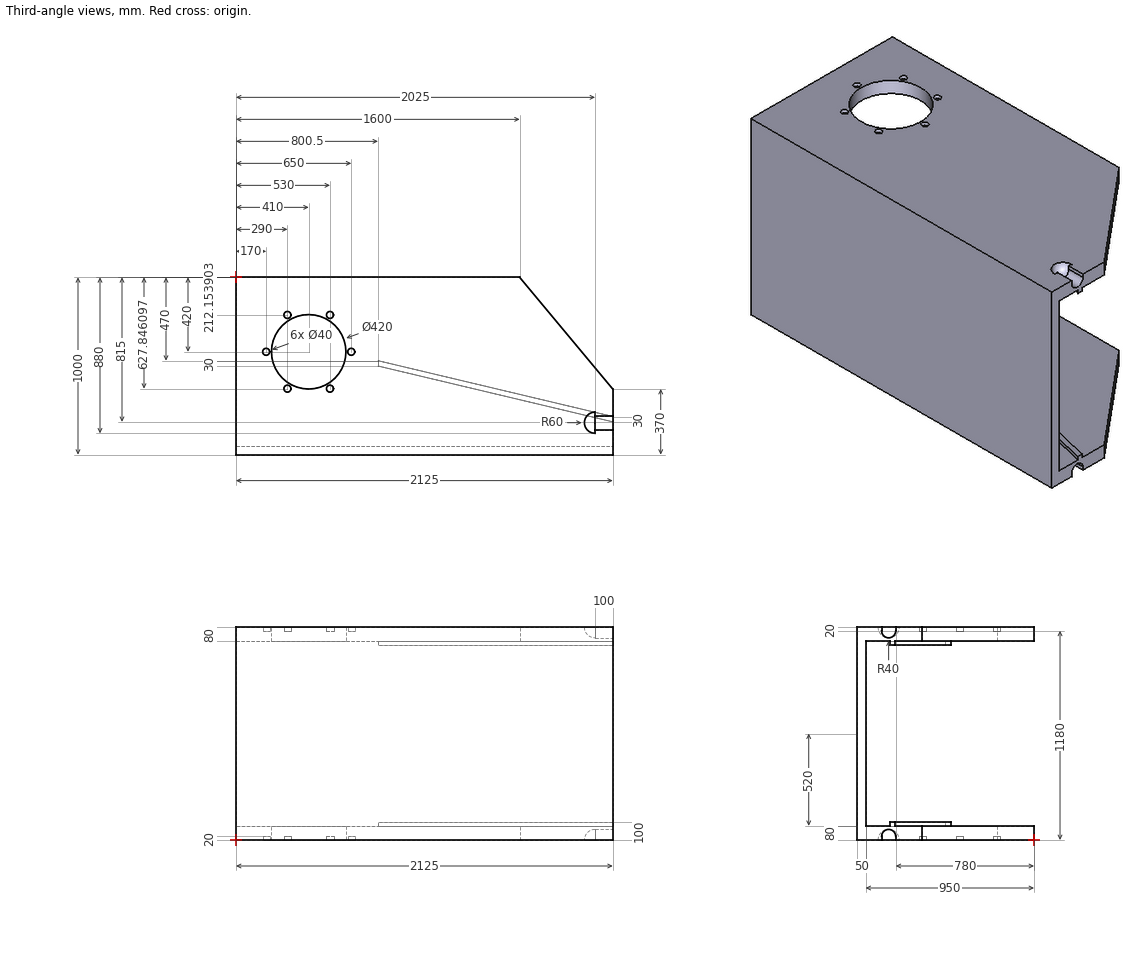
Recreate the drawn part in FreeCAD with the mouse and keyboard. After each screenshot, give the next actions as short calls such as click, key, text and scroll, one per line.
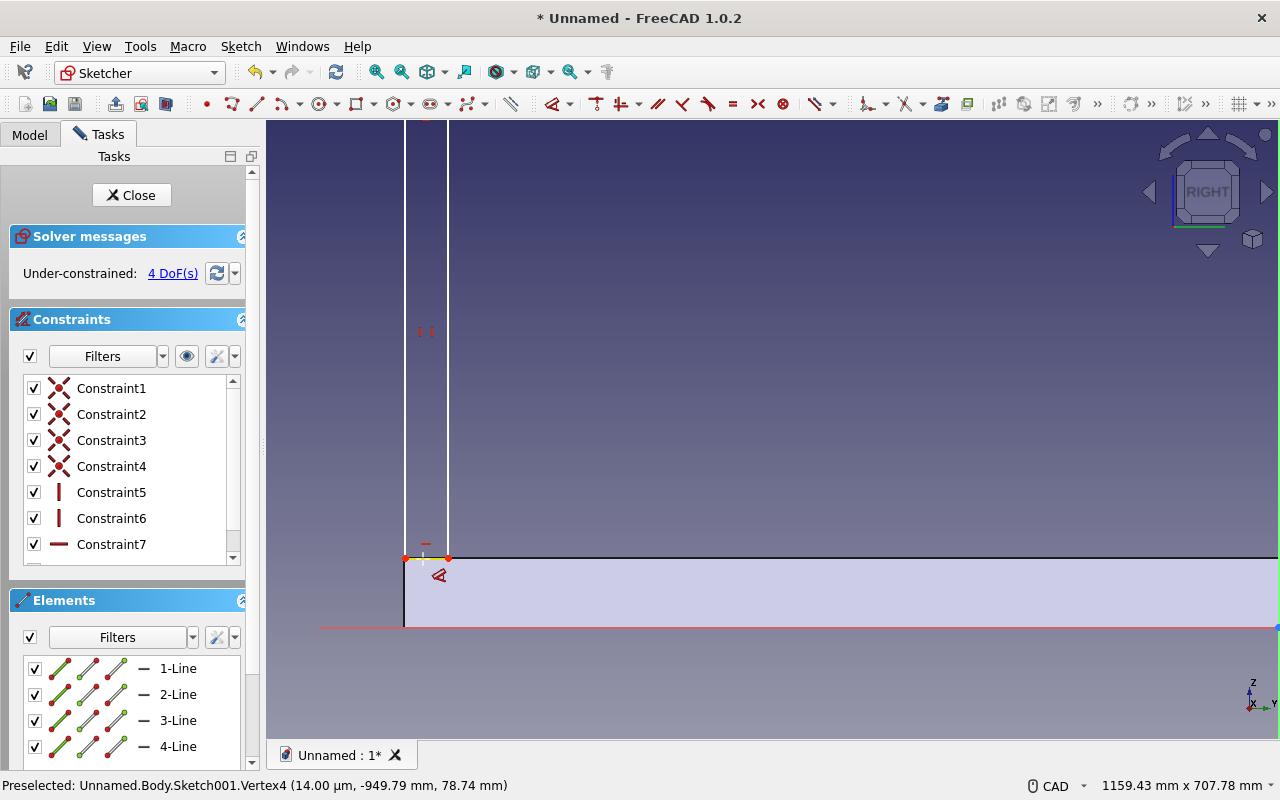
click(422, 559)
click(427, 593)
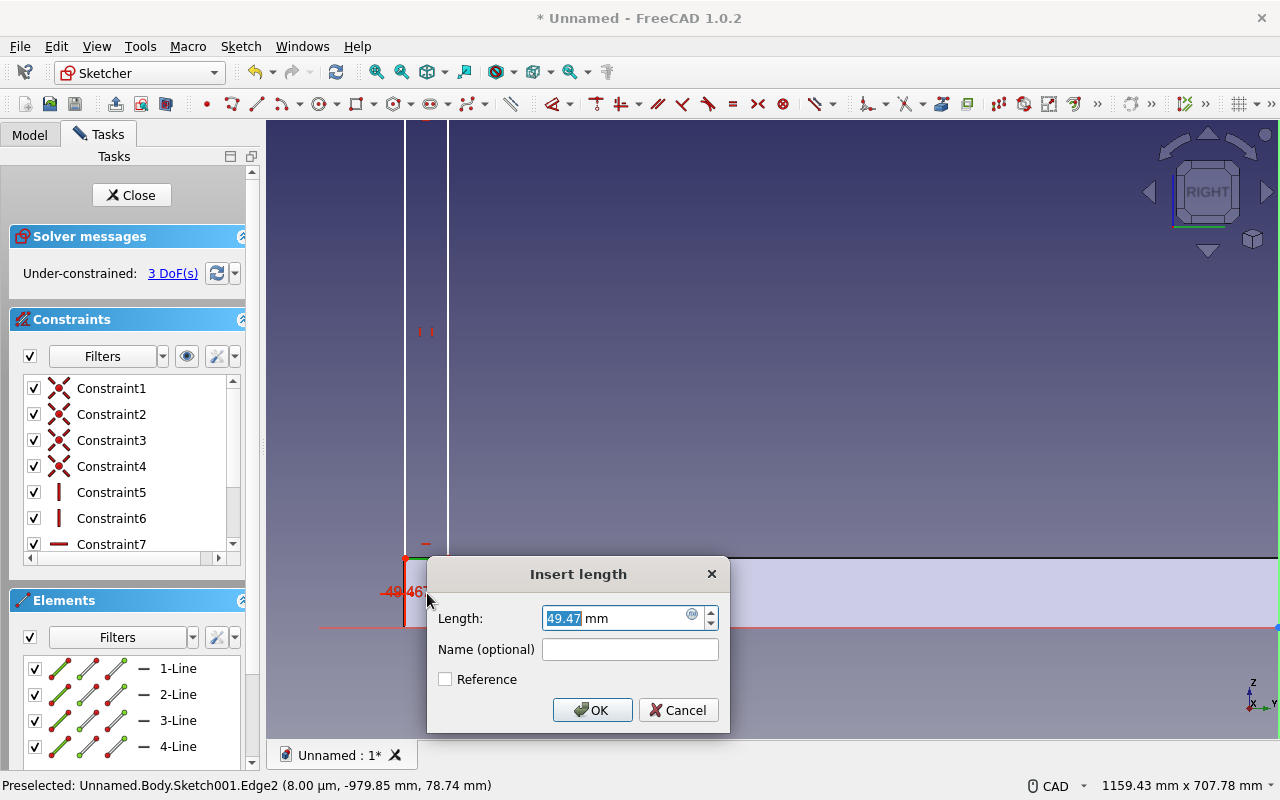
text(50)
key(Return)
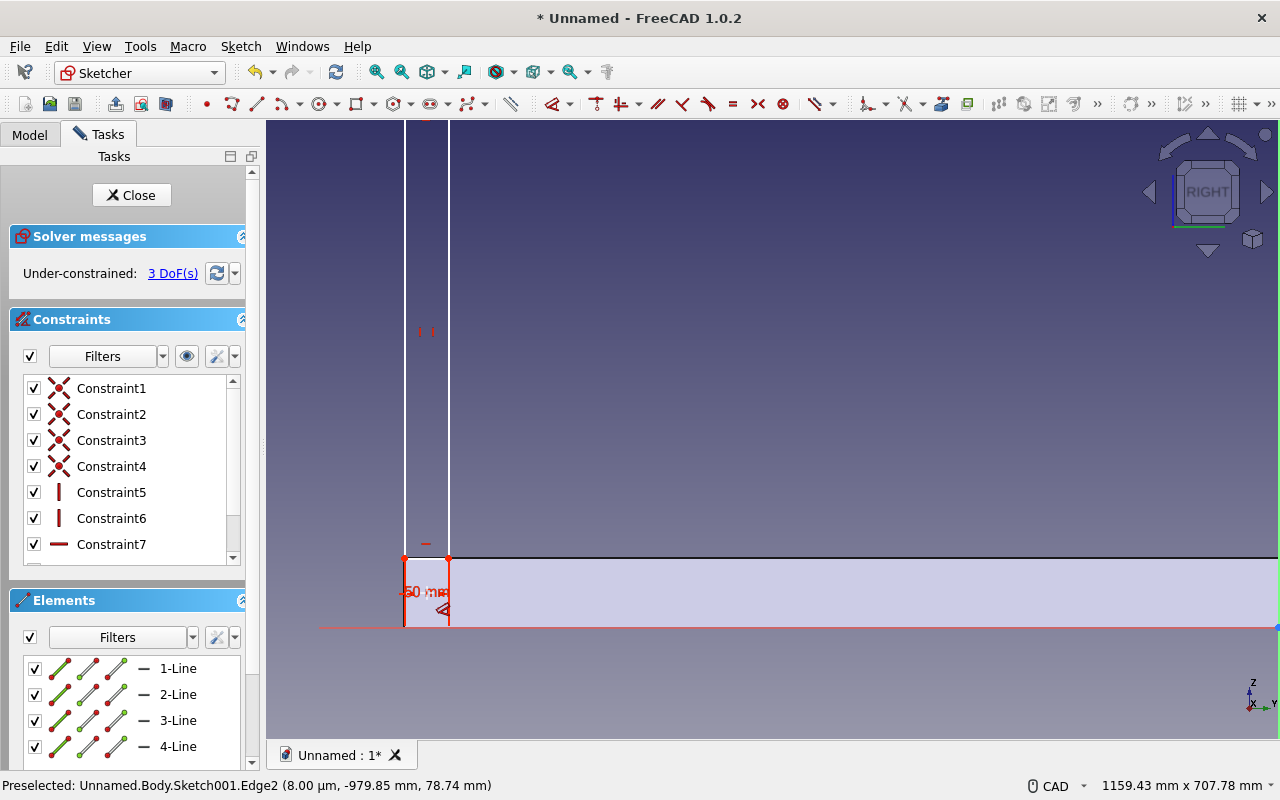
click(405, 240)
click(371, 353)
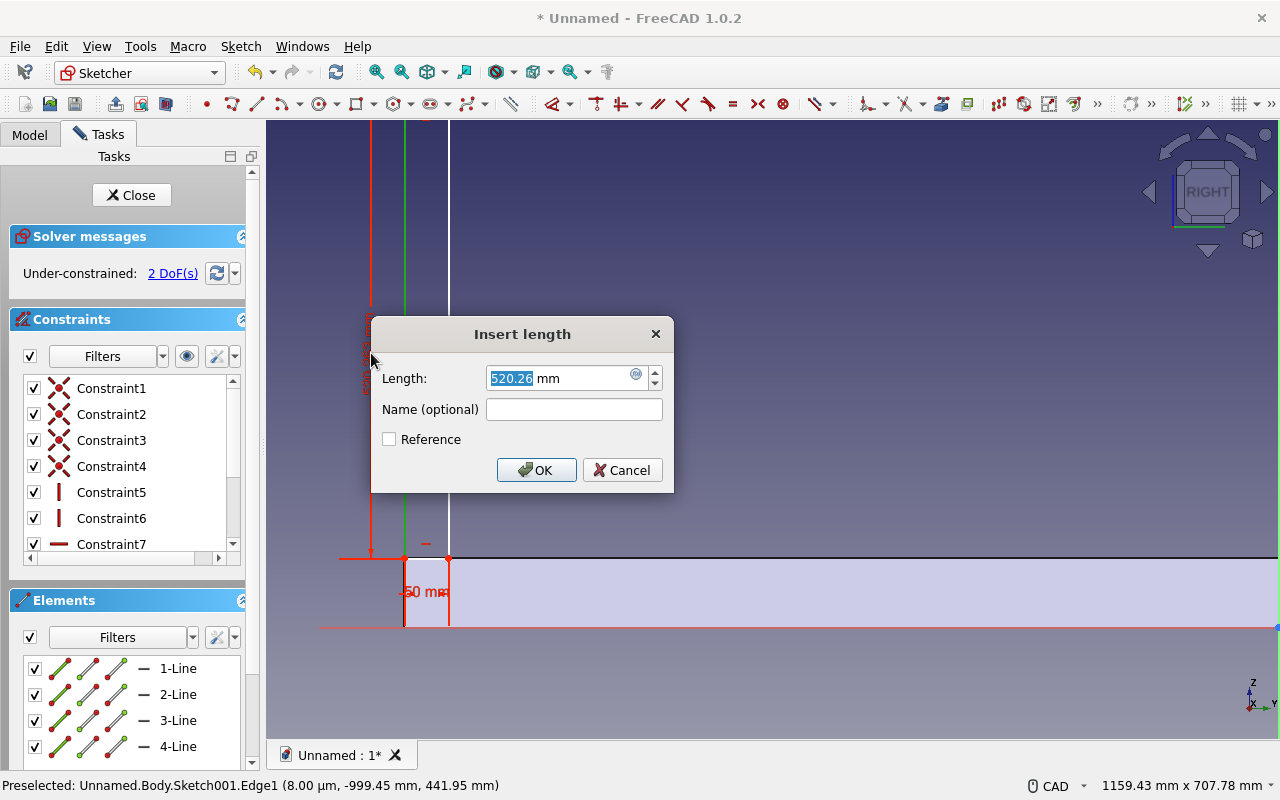
text(520)
key(Return)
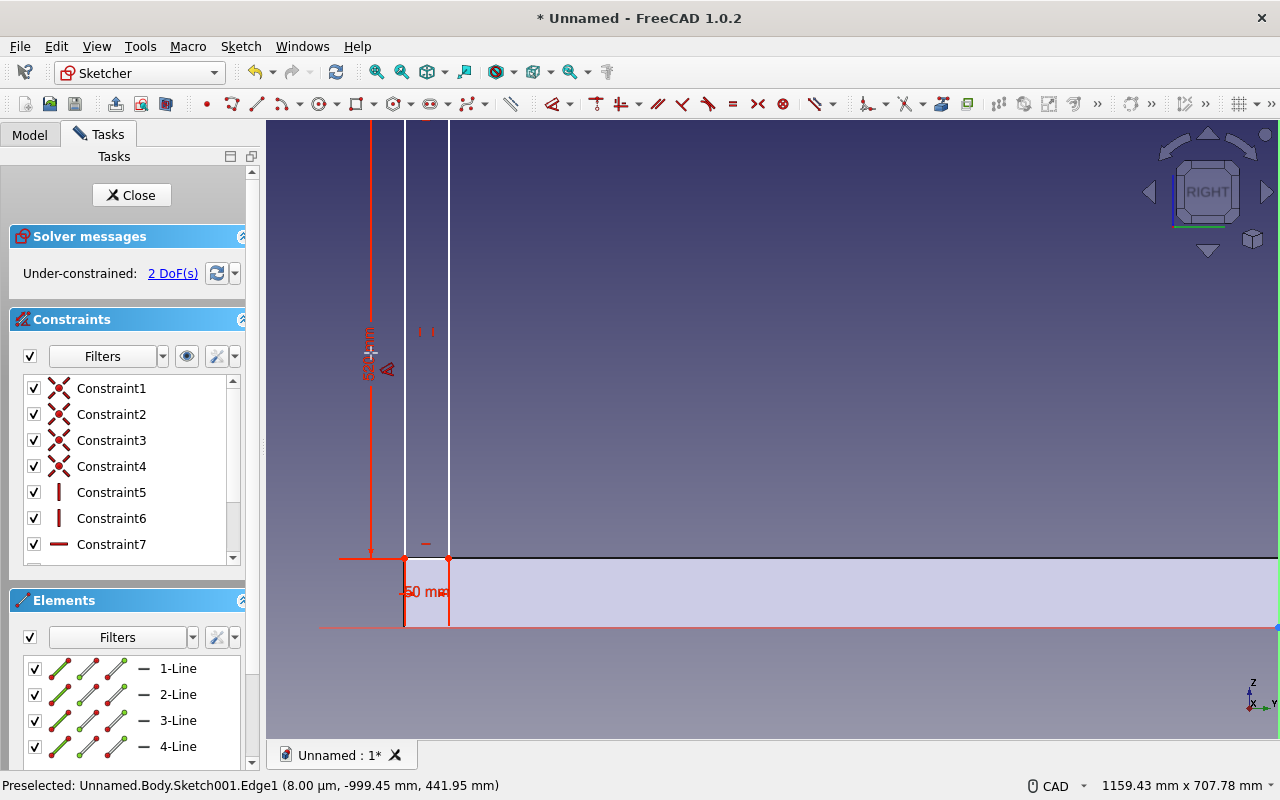
click(405, 559)
click(371, 569)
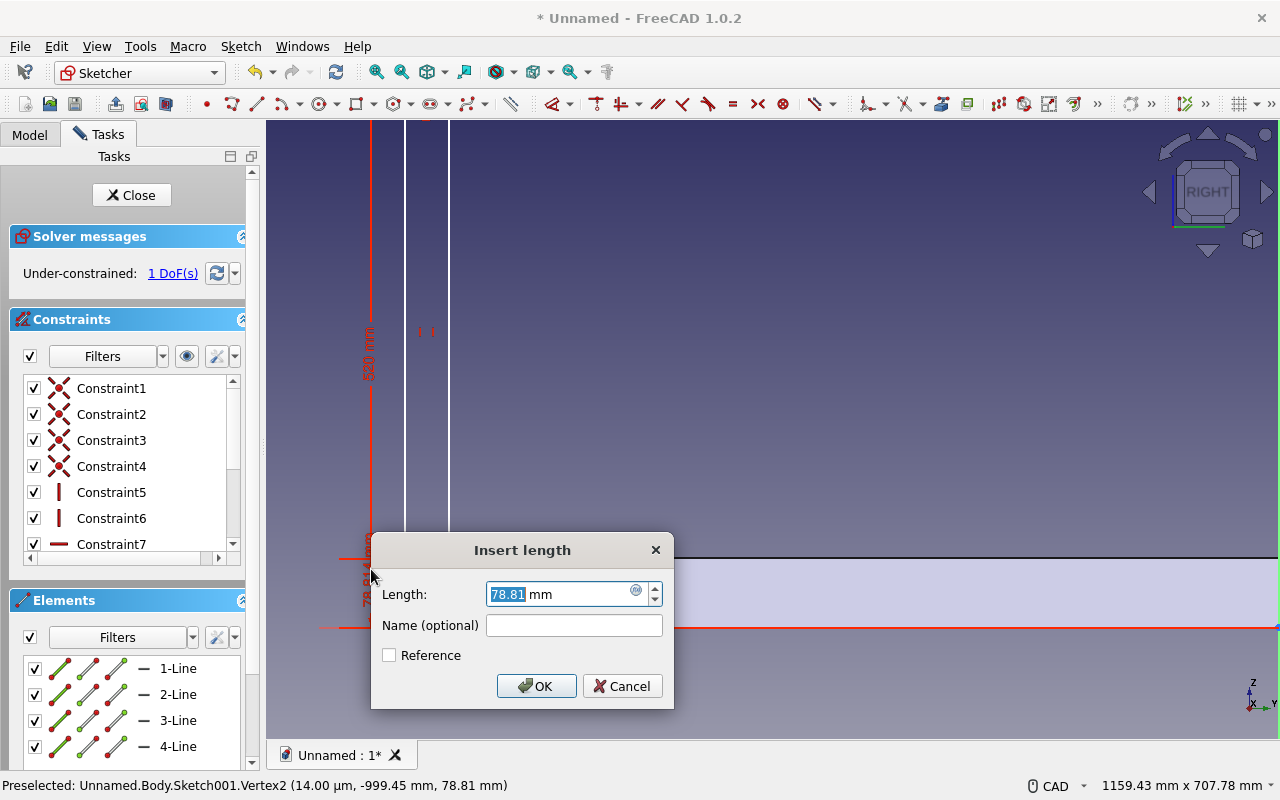
text(80)
key(Return)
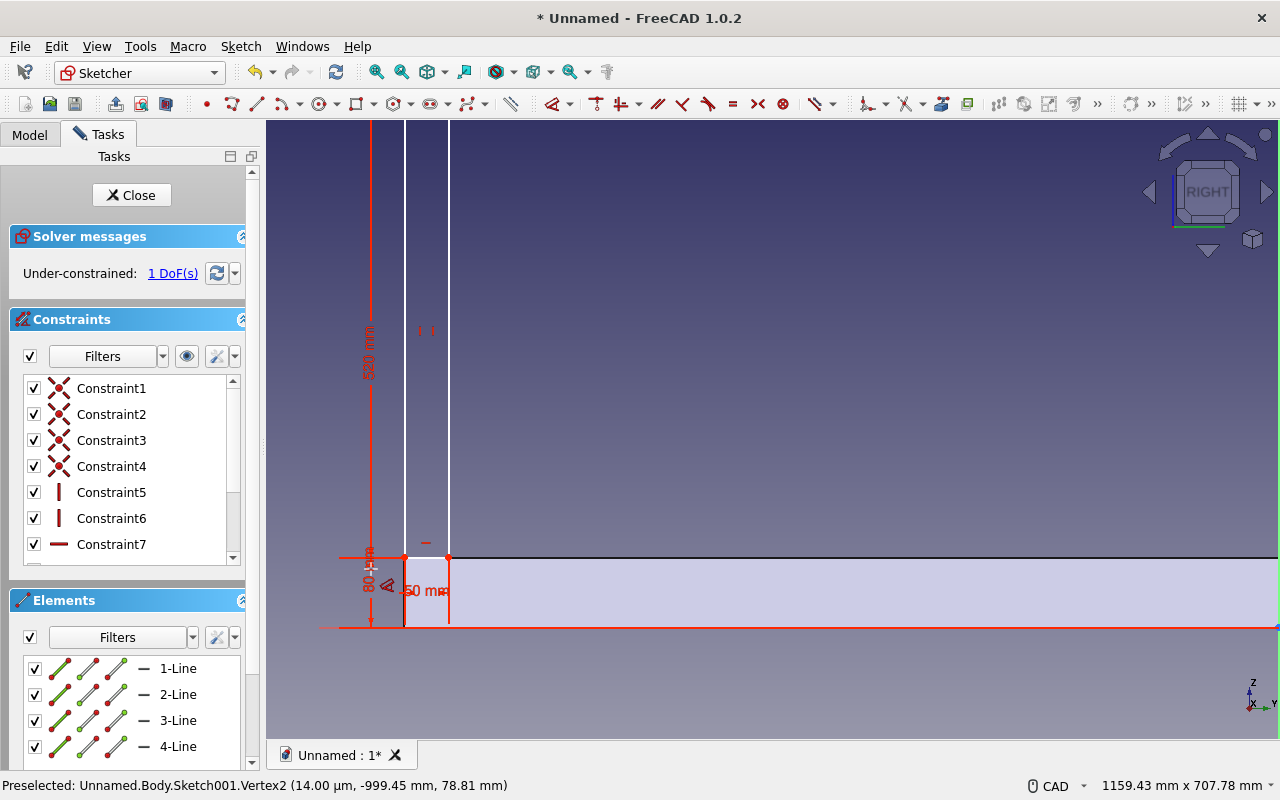
click(449, 558)
click(782, 662)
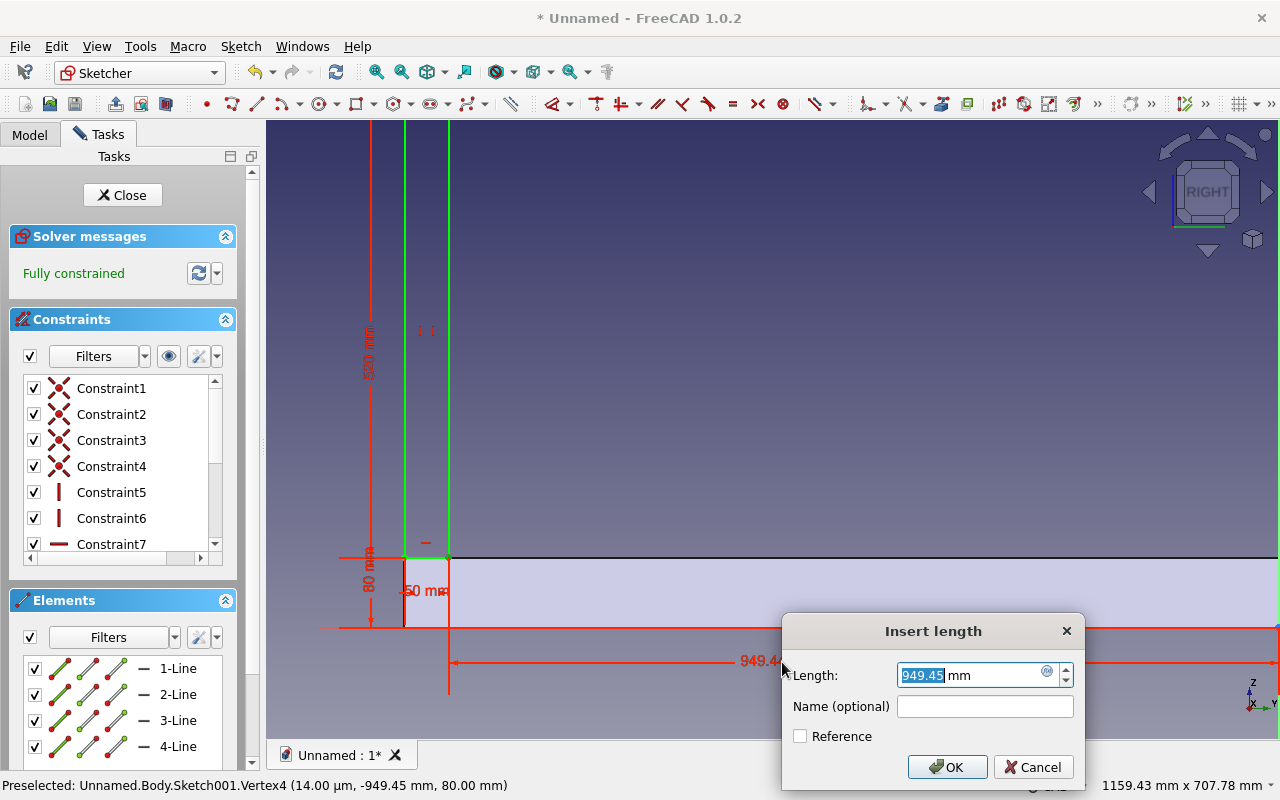
text(950)
key(Return)
key(Escape)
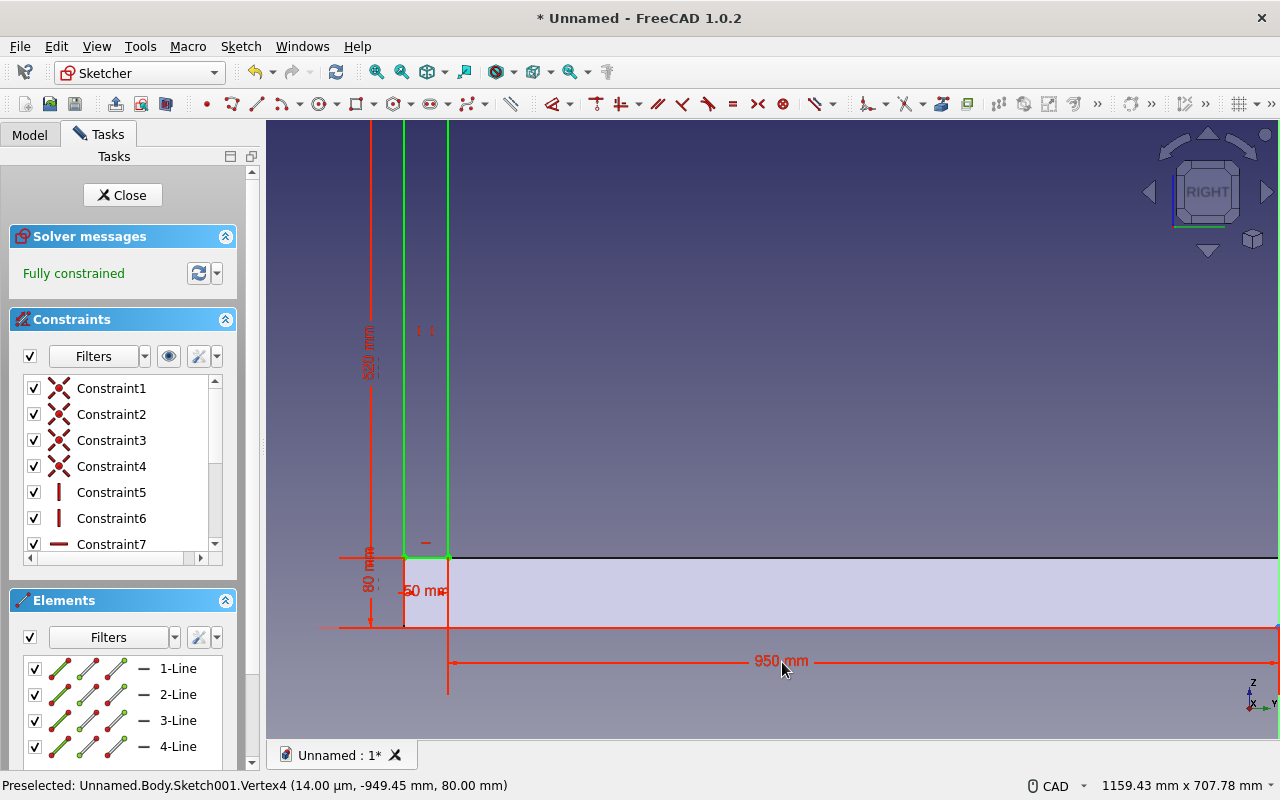
click(123, 195)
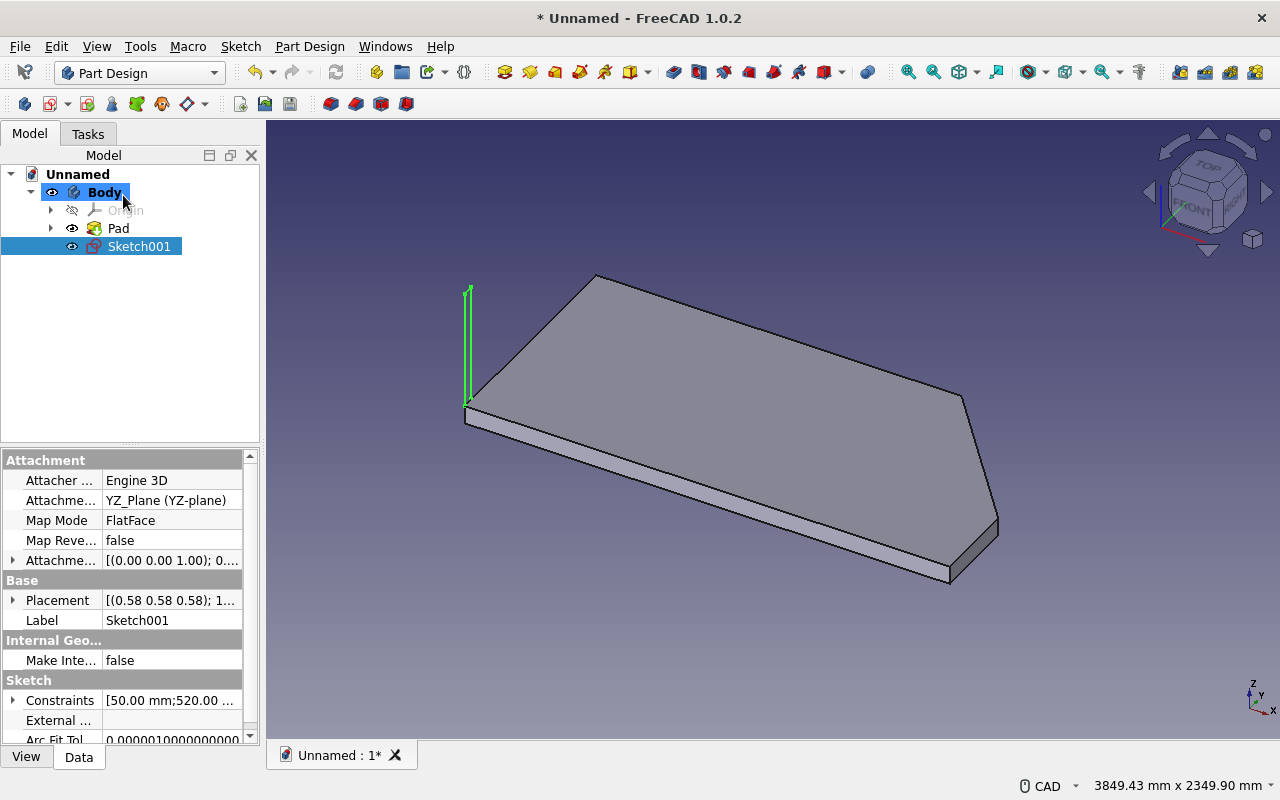
click(505, 72)